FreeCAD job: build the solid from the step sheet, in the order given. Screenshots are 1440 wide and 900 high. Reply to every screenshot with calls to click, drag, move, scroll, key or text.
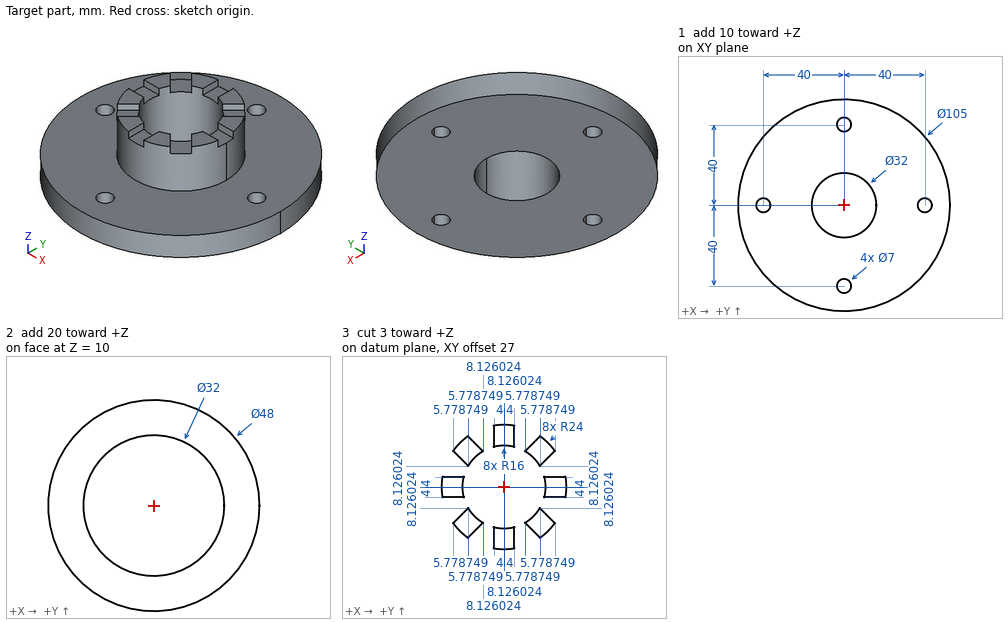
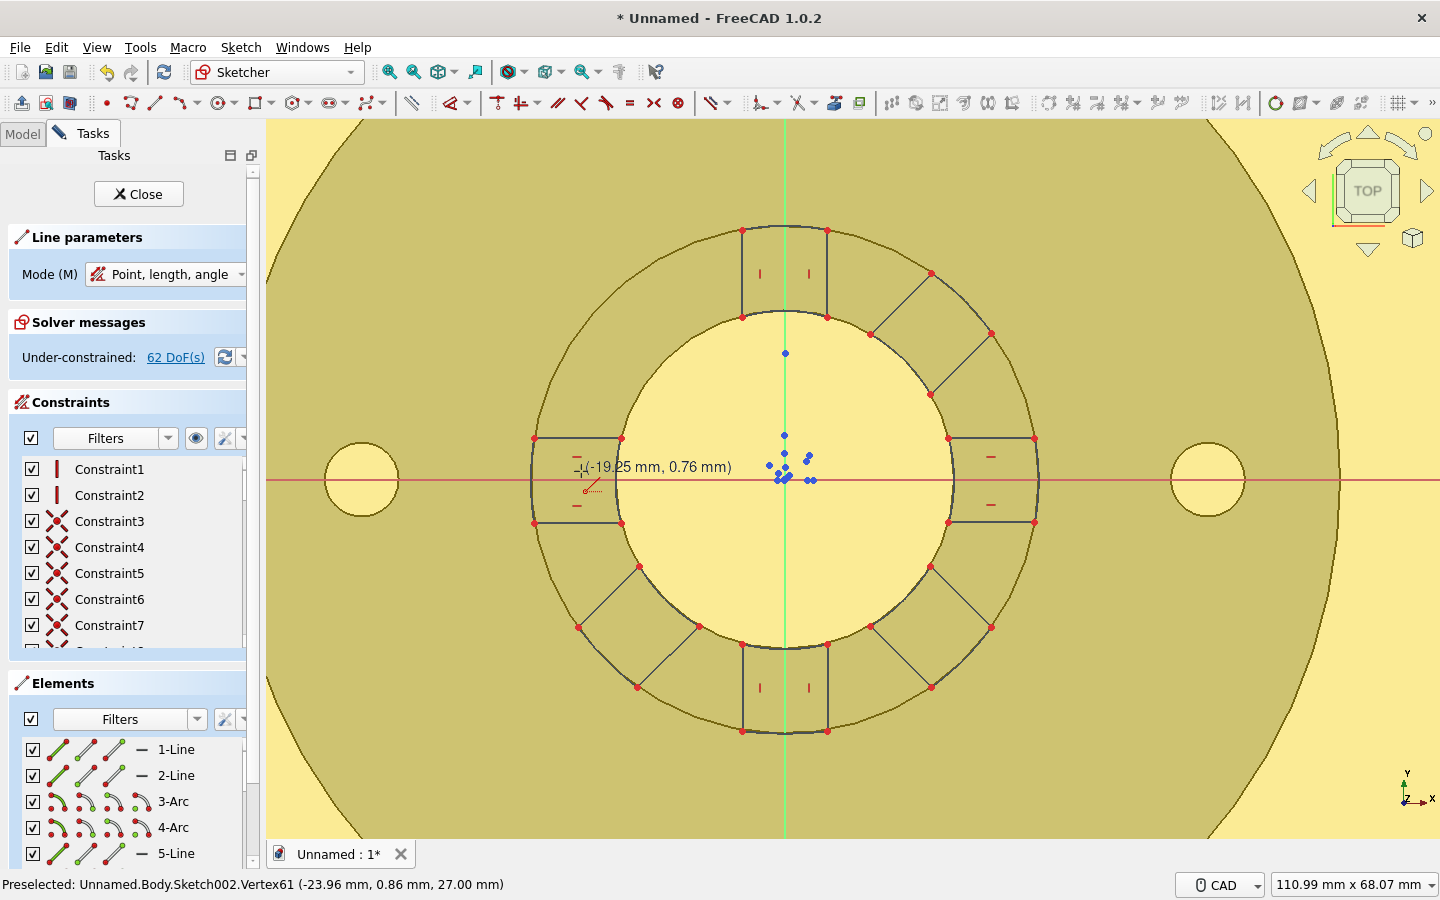
click(578, 333)
click(639, 394)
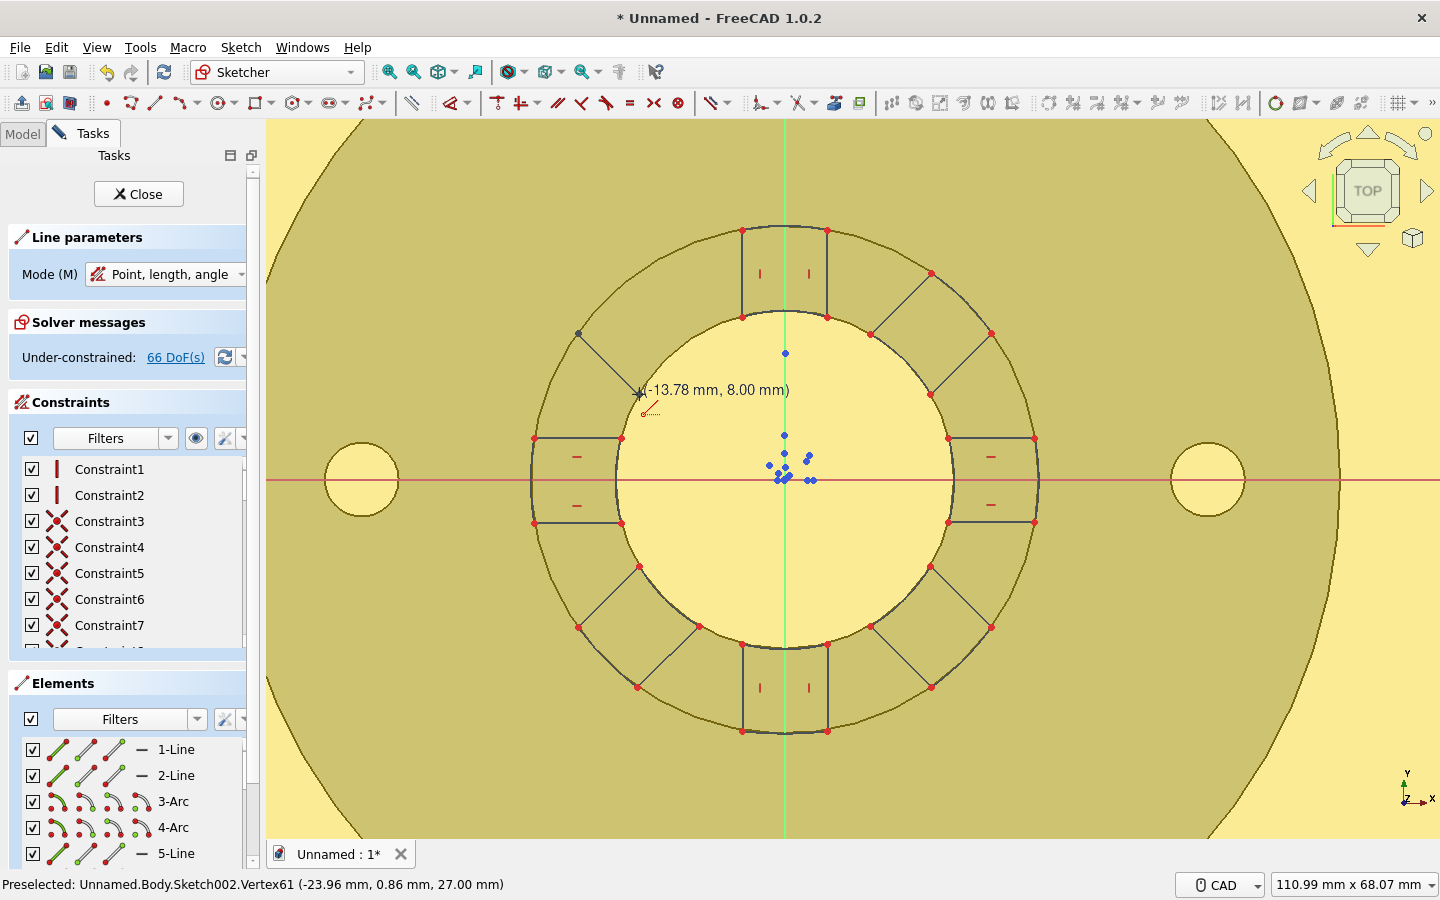
click(699, 334)
click(638, 273)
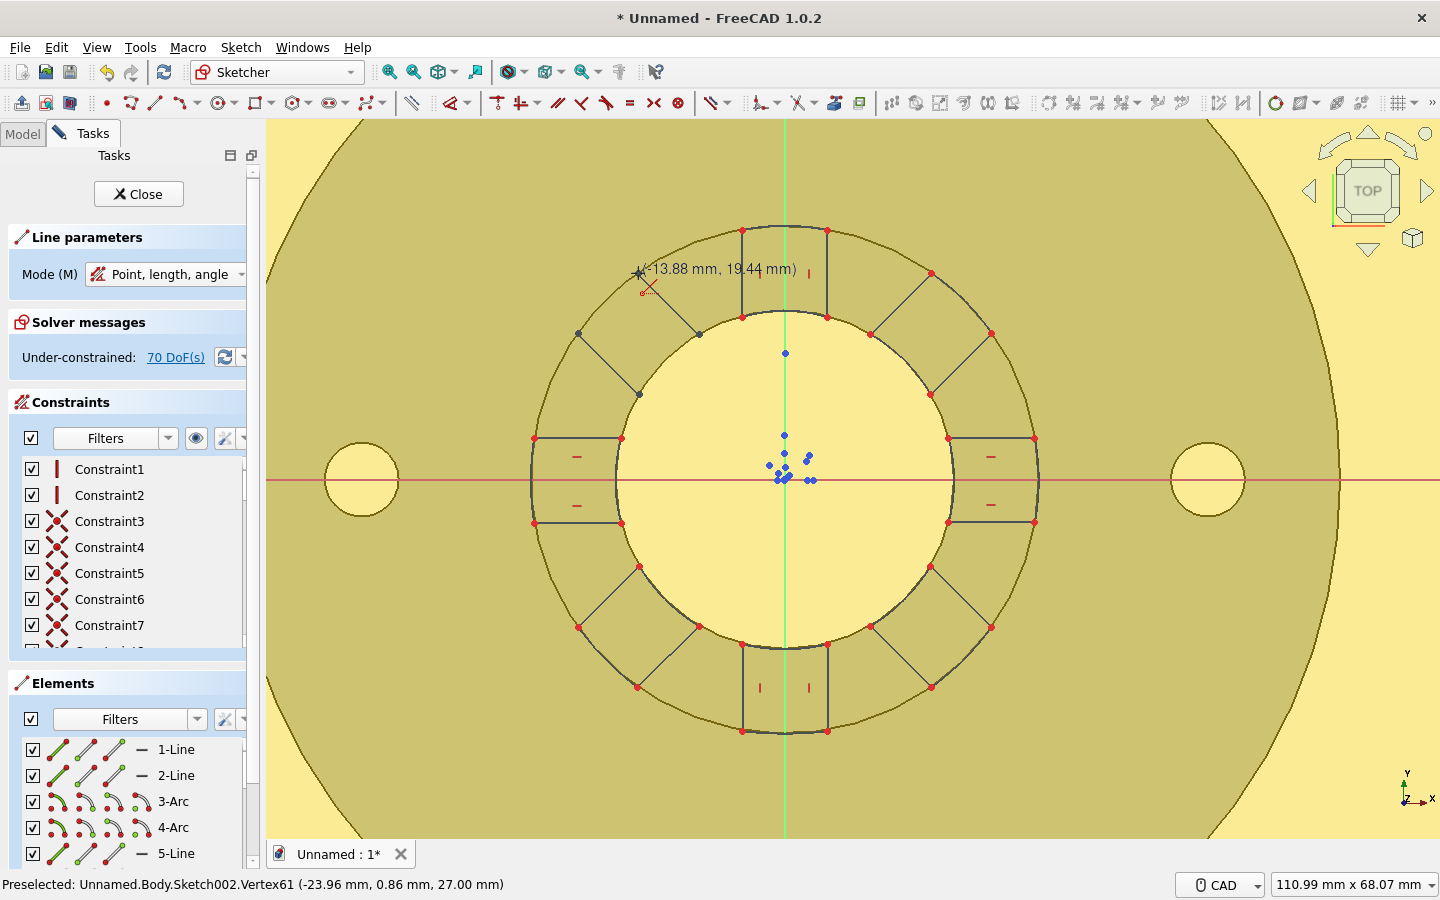
click(180, 104)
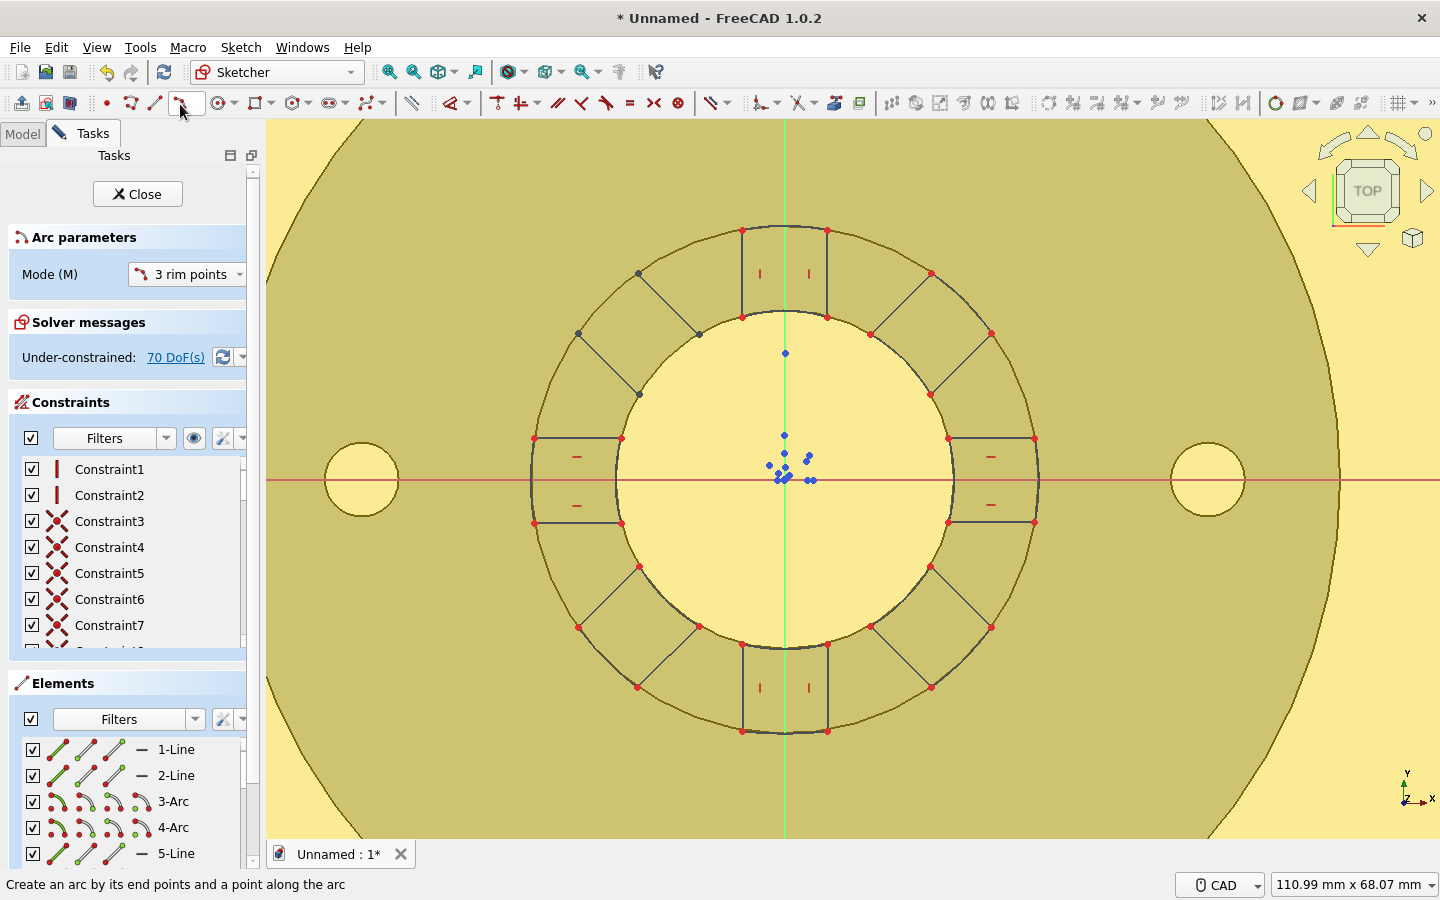
click(639, 395)
click(699, 335)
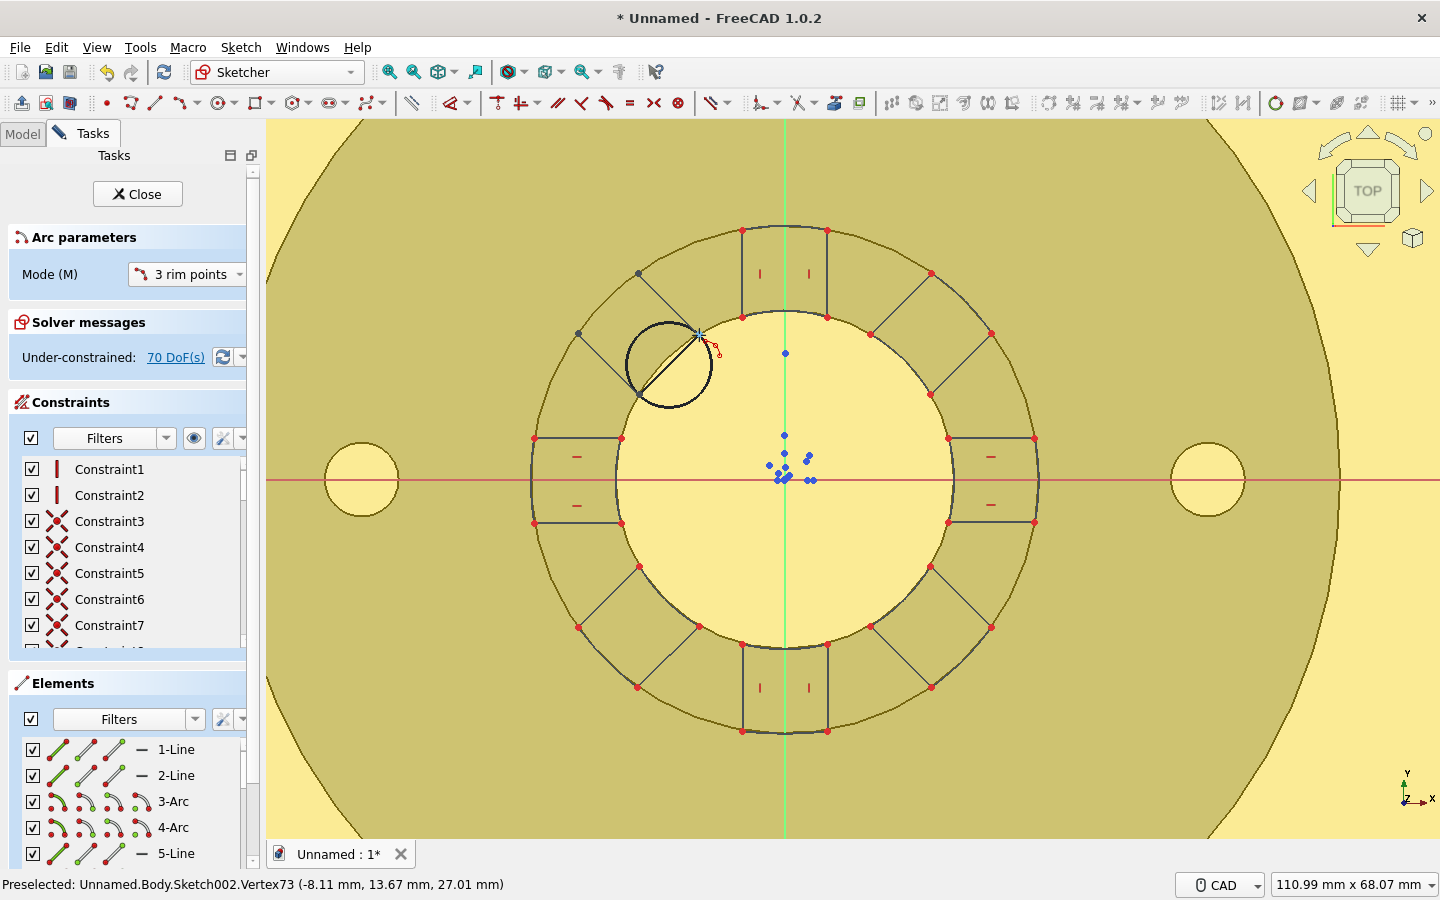
scroll(665, 360, up, 6)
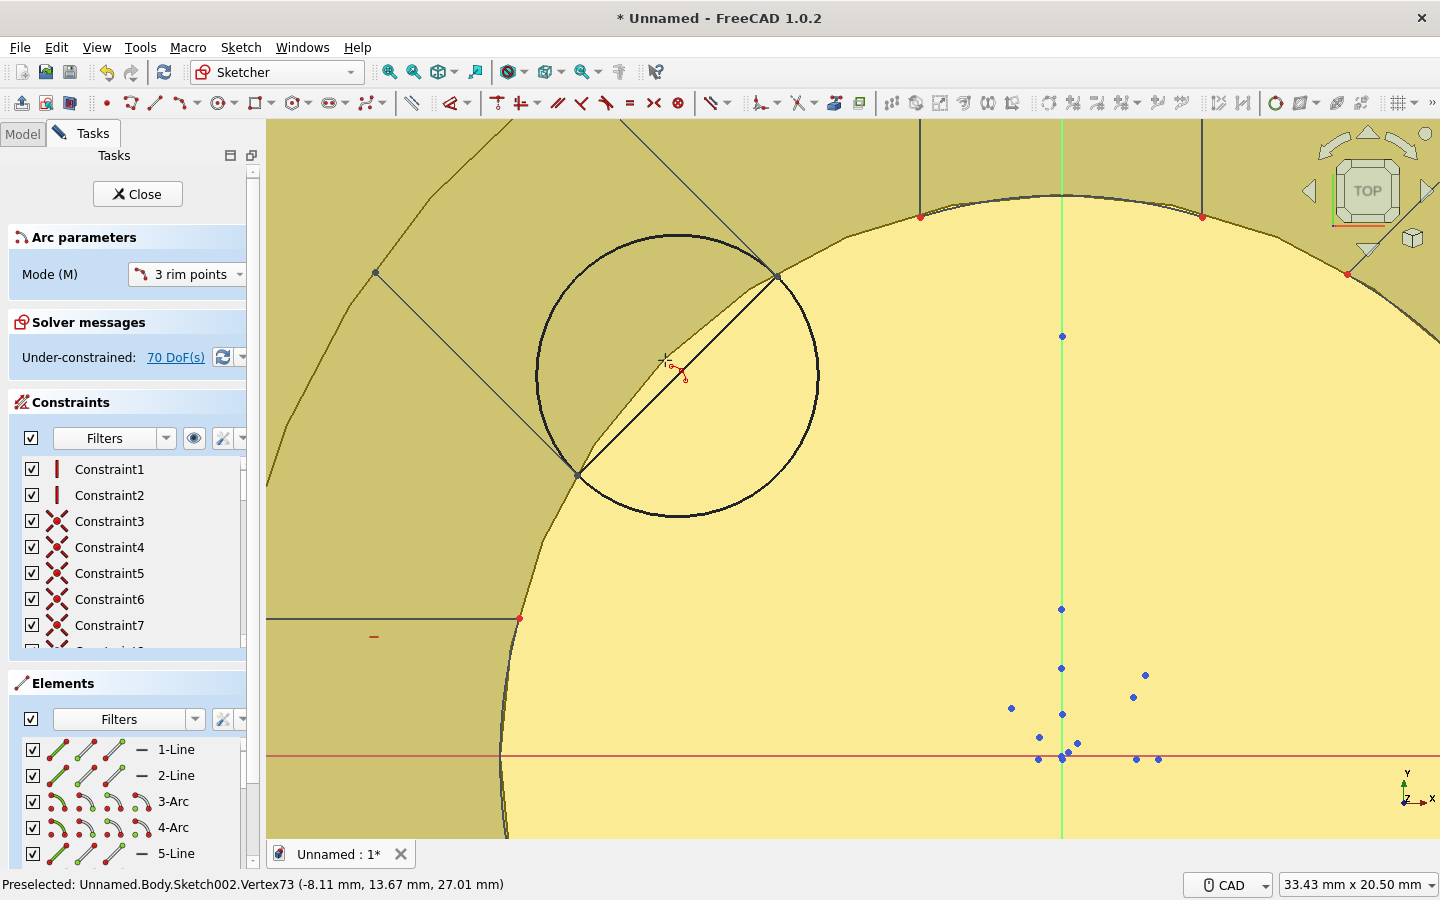
click(665, 359)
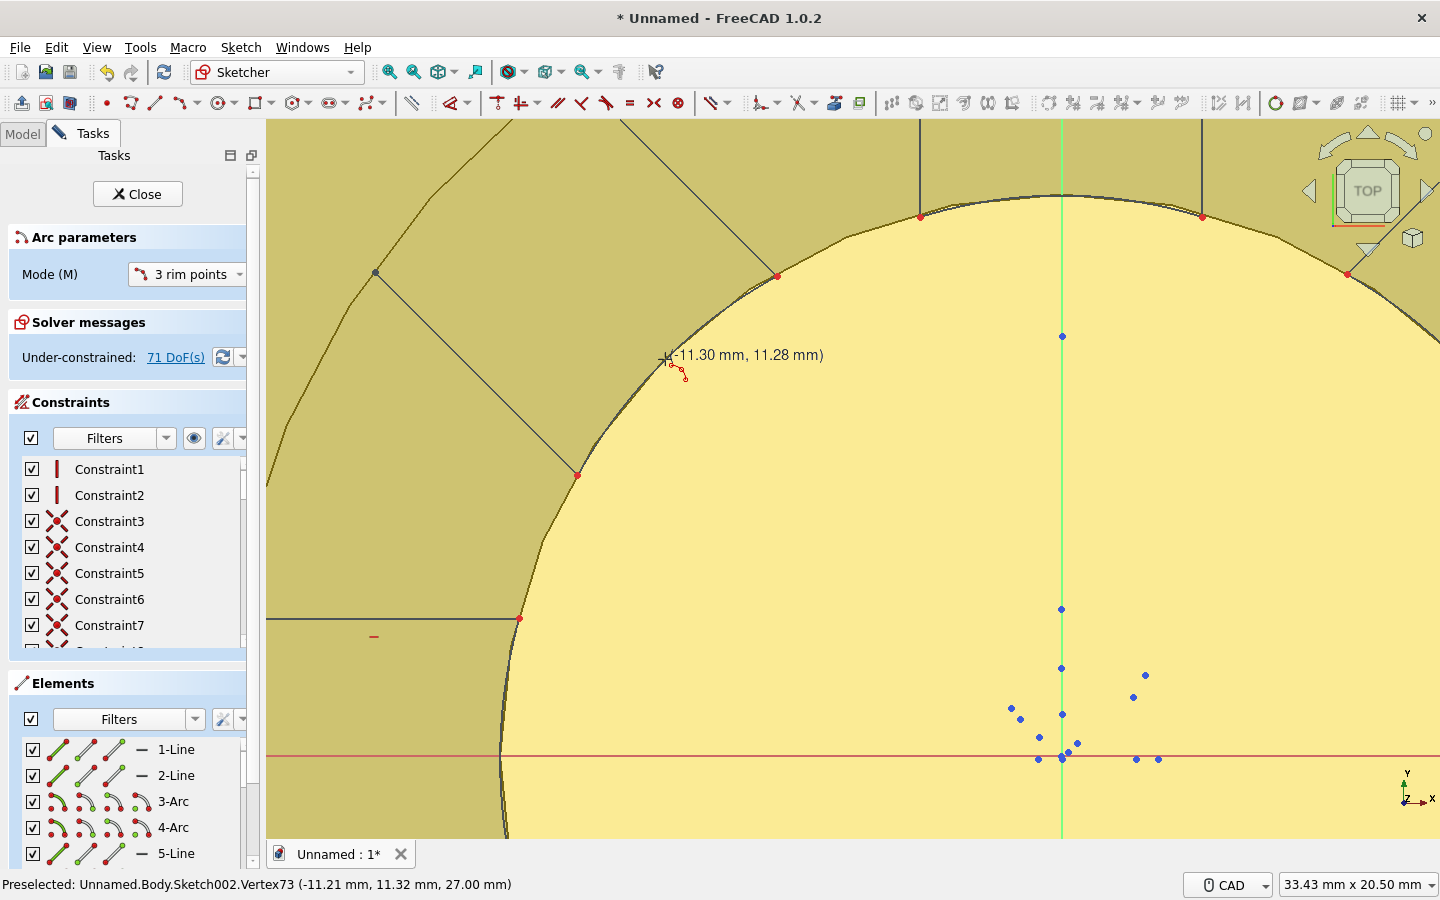
scroll(665, 360, down, 6)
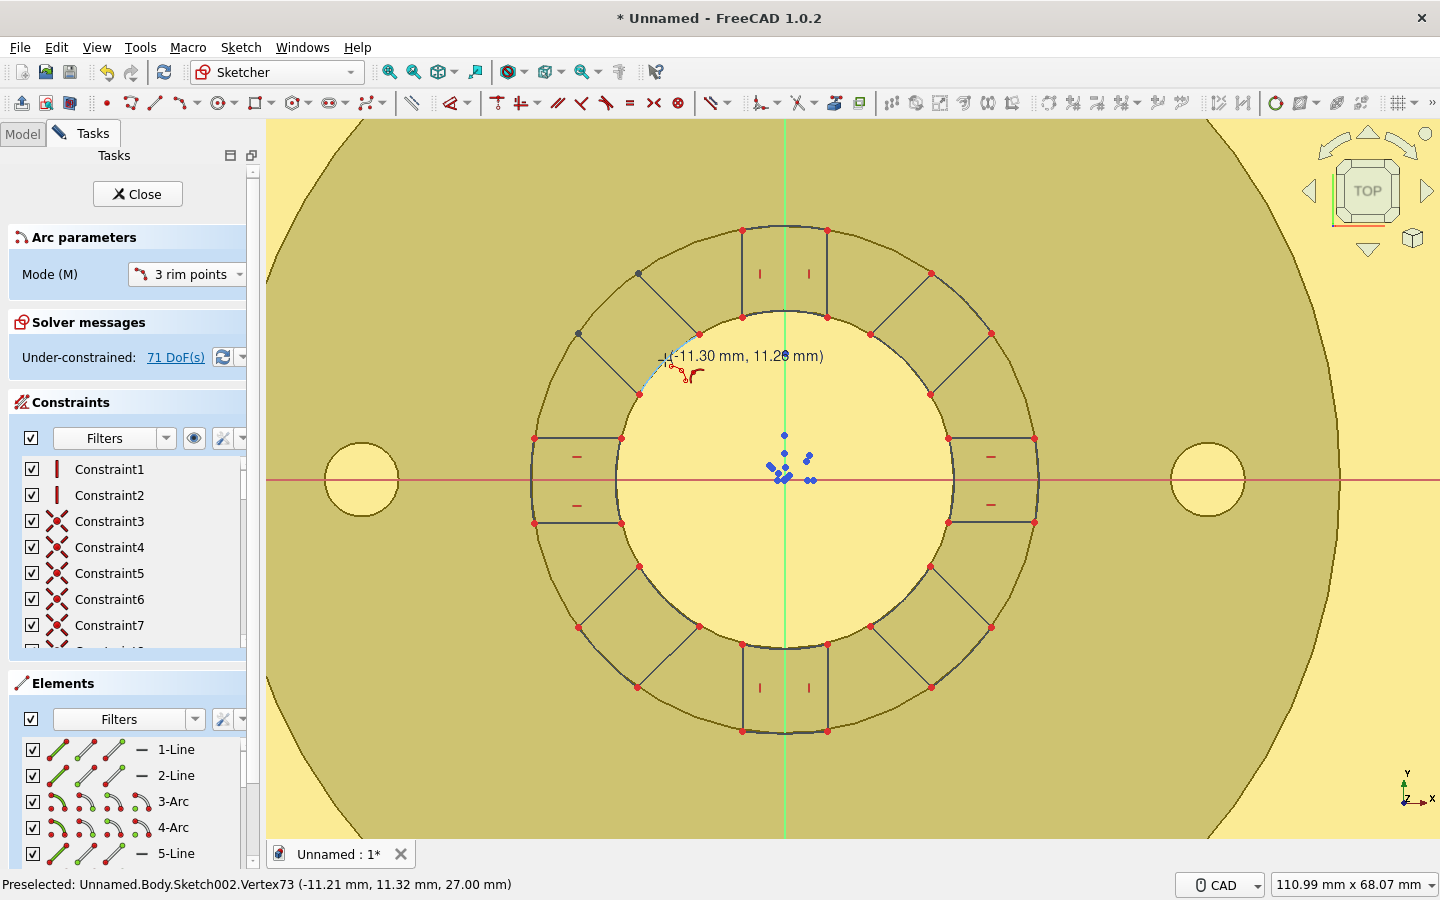
click(638, 274)
click(578, 334)